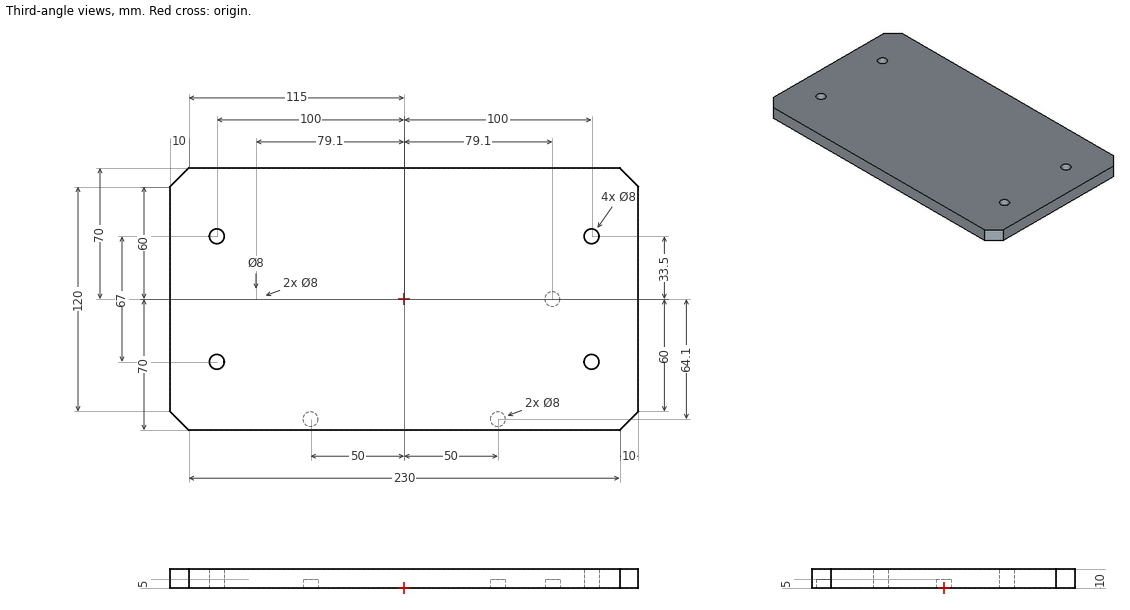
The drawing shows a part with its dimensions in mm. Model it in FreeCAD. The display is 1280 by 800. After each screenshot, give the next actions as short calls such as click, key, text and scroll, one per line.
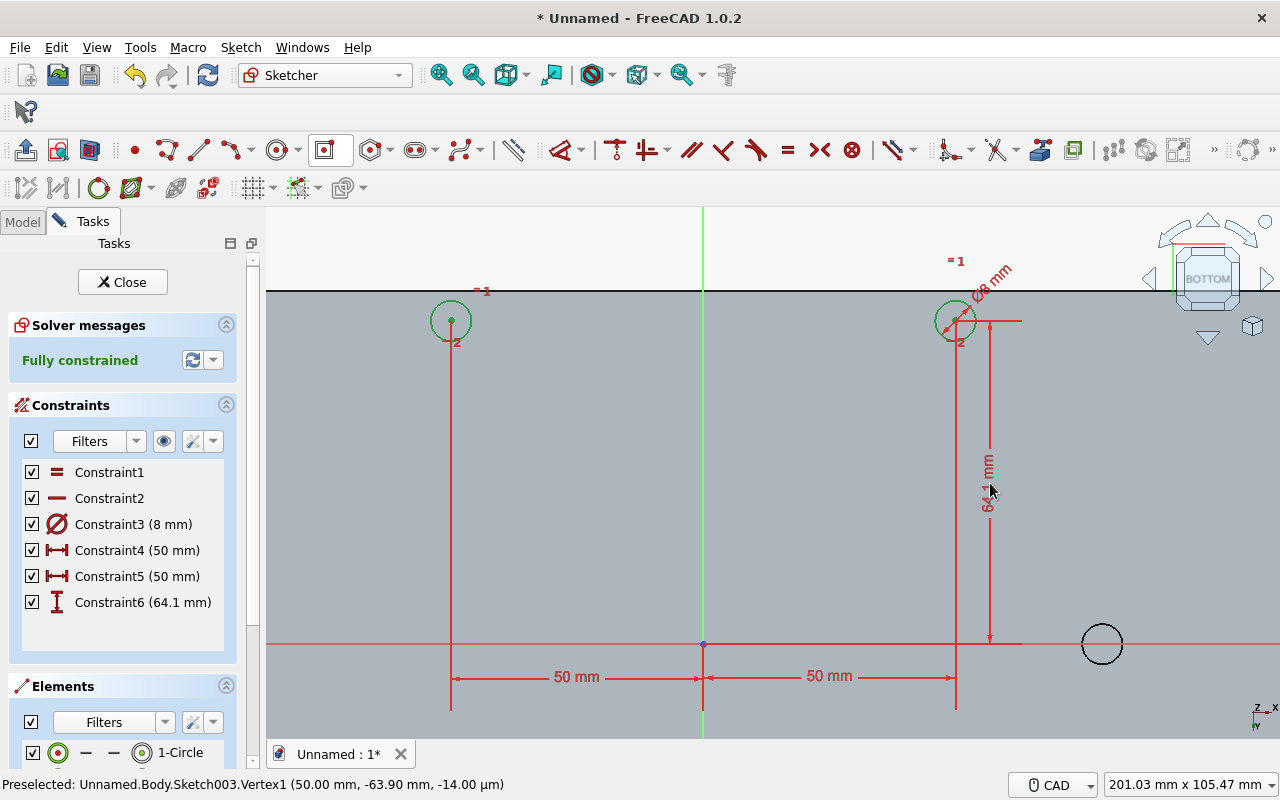
click(123, 282)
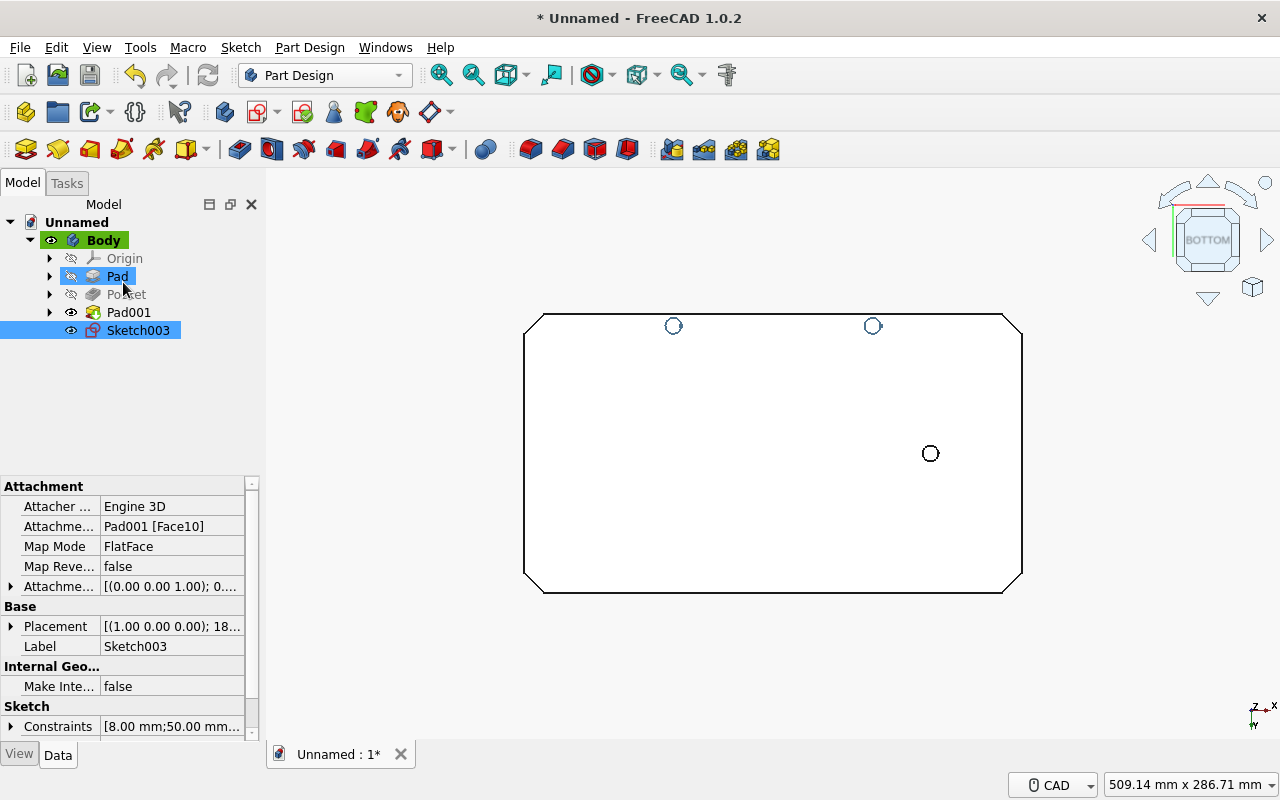
click(240, 150)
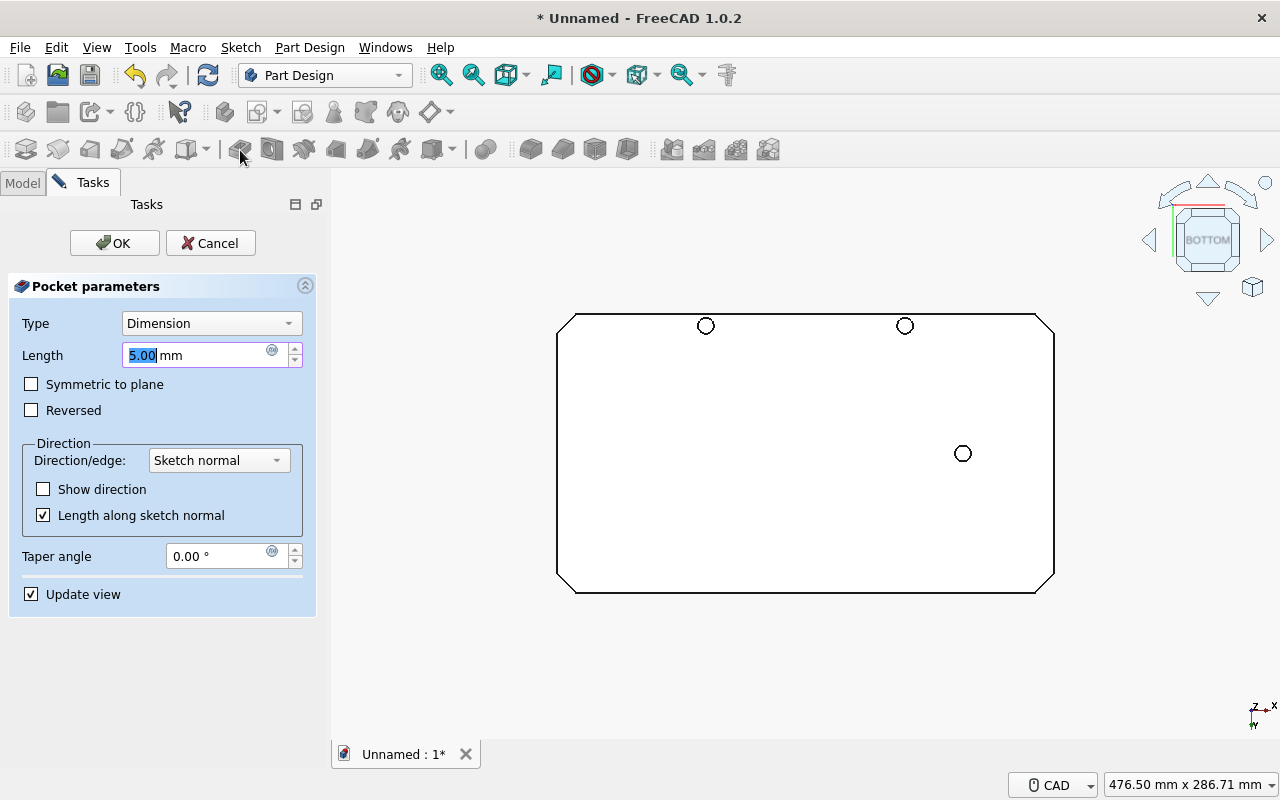
text(5)
key(Tab)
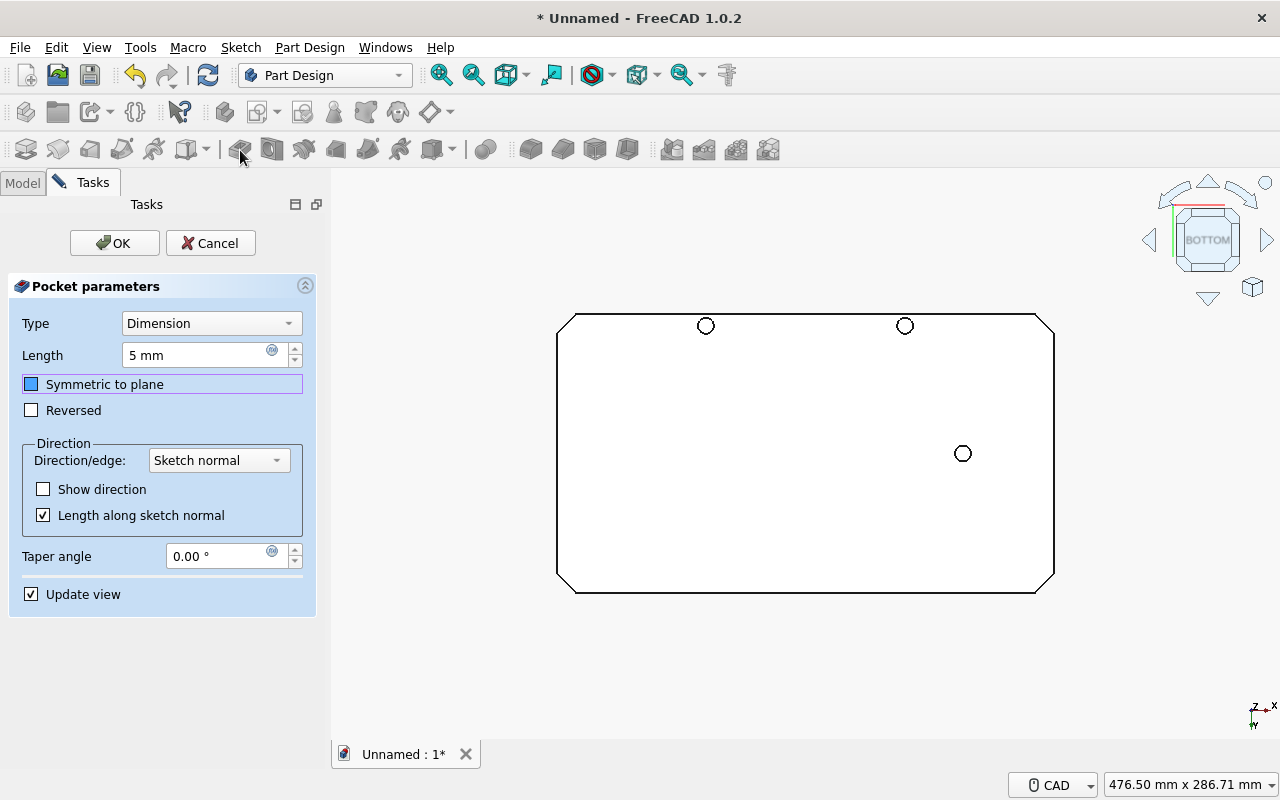
click(115, 243)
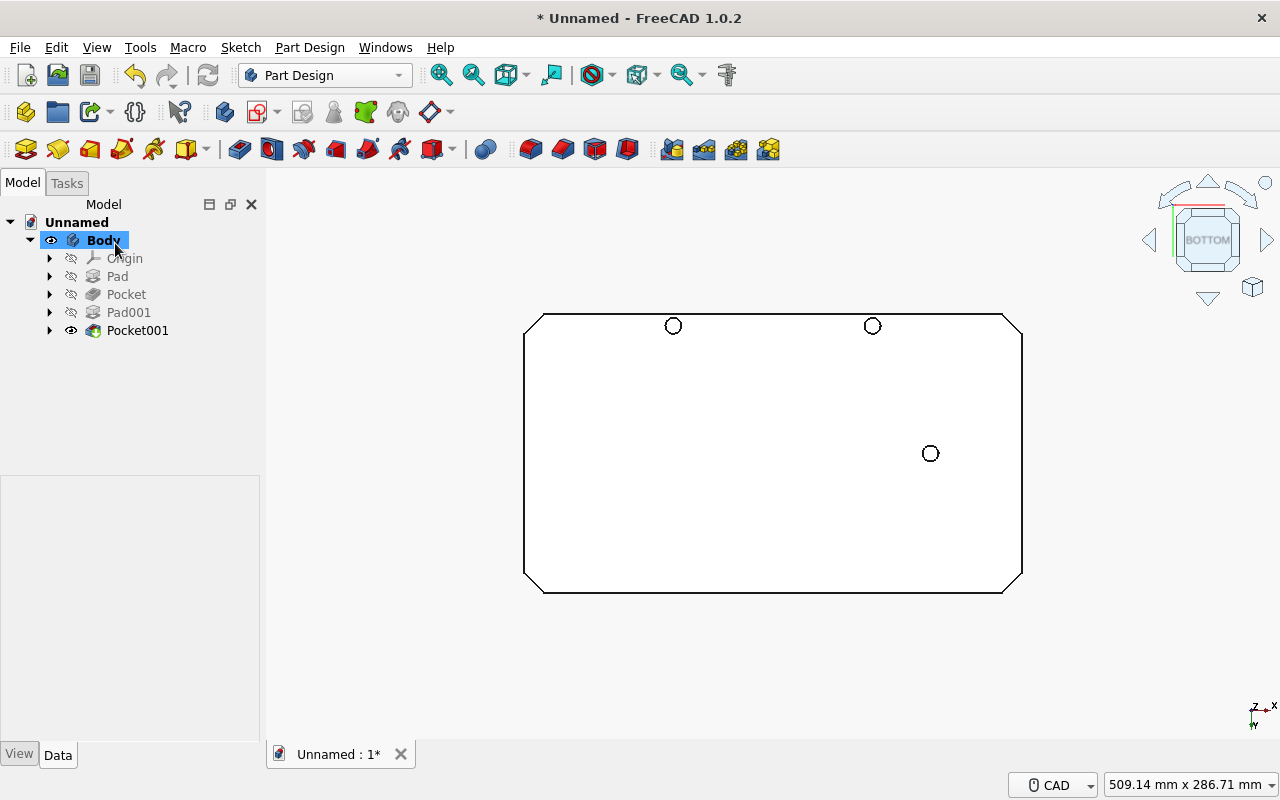
key(0)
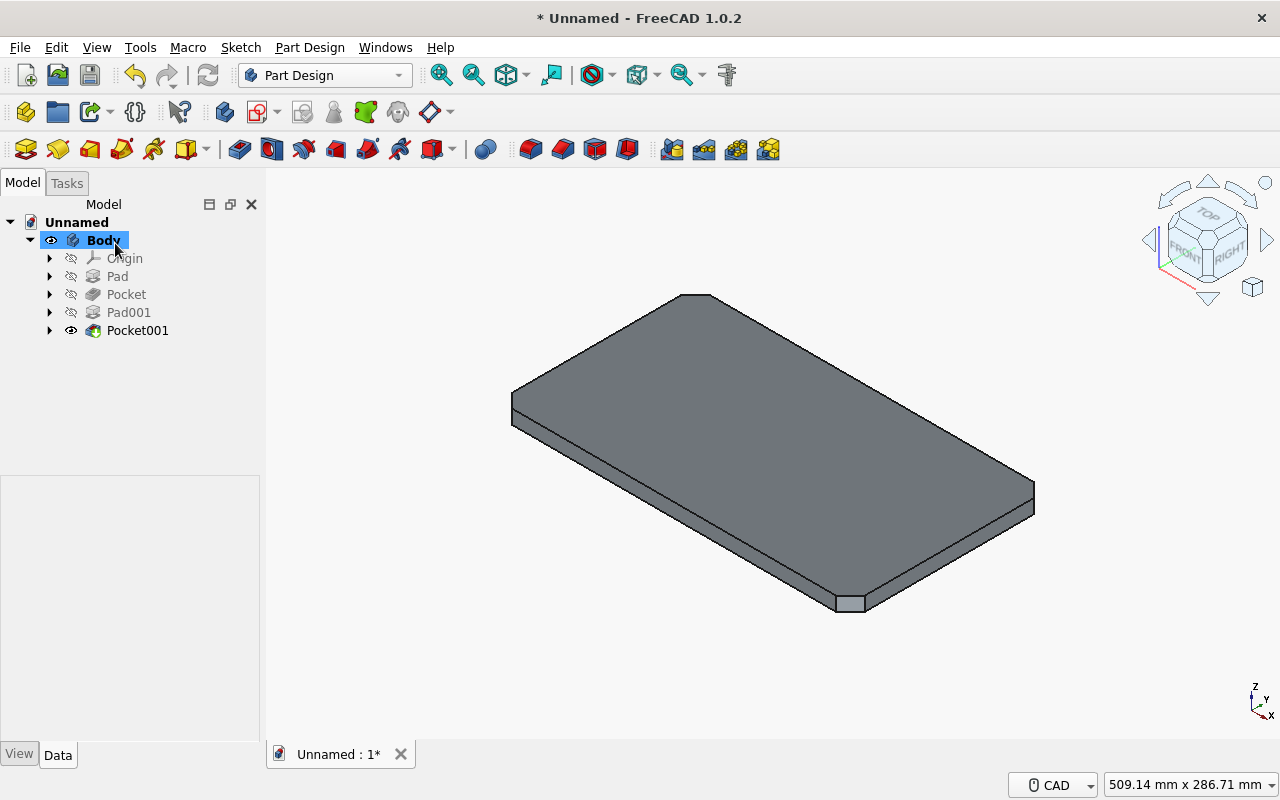
click(823, 473)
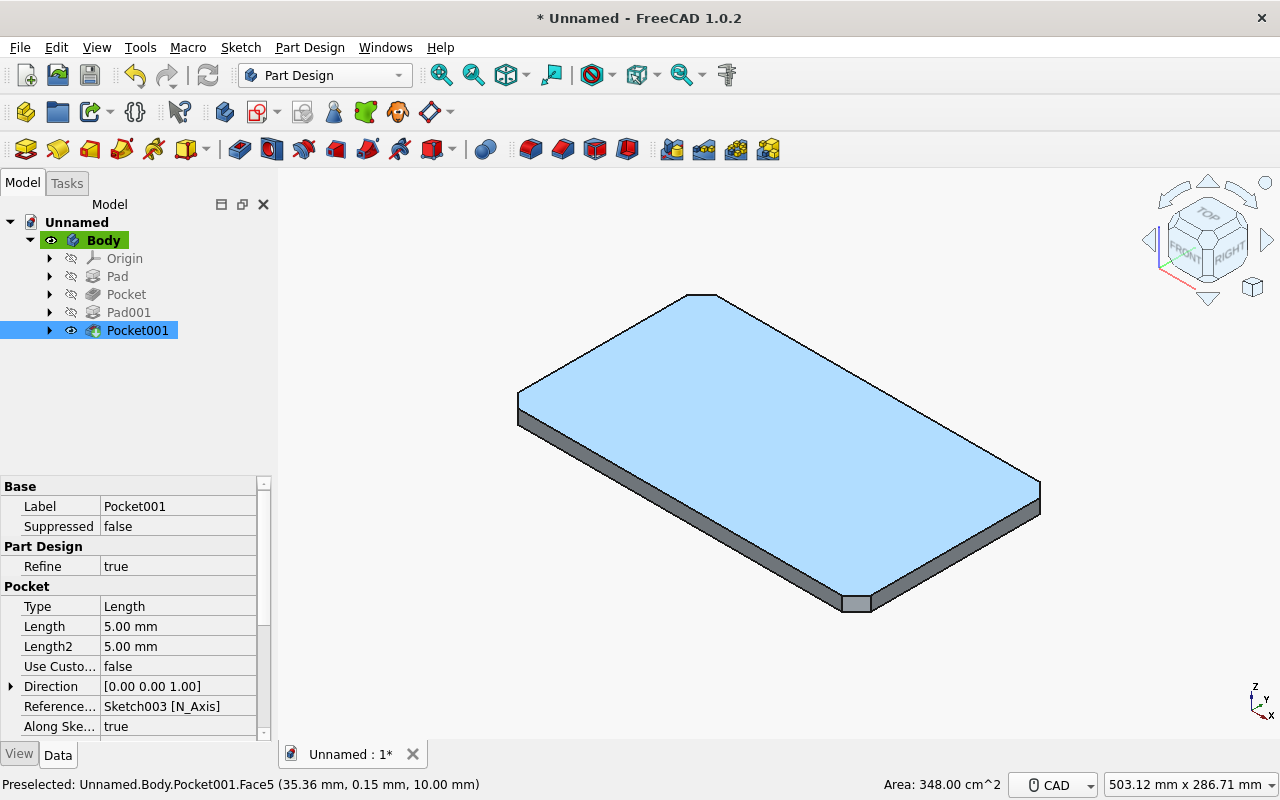
click(258, 112)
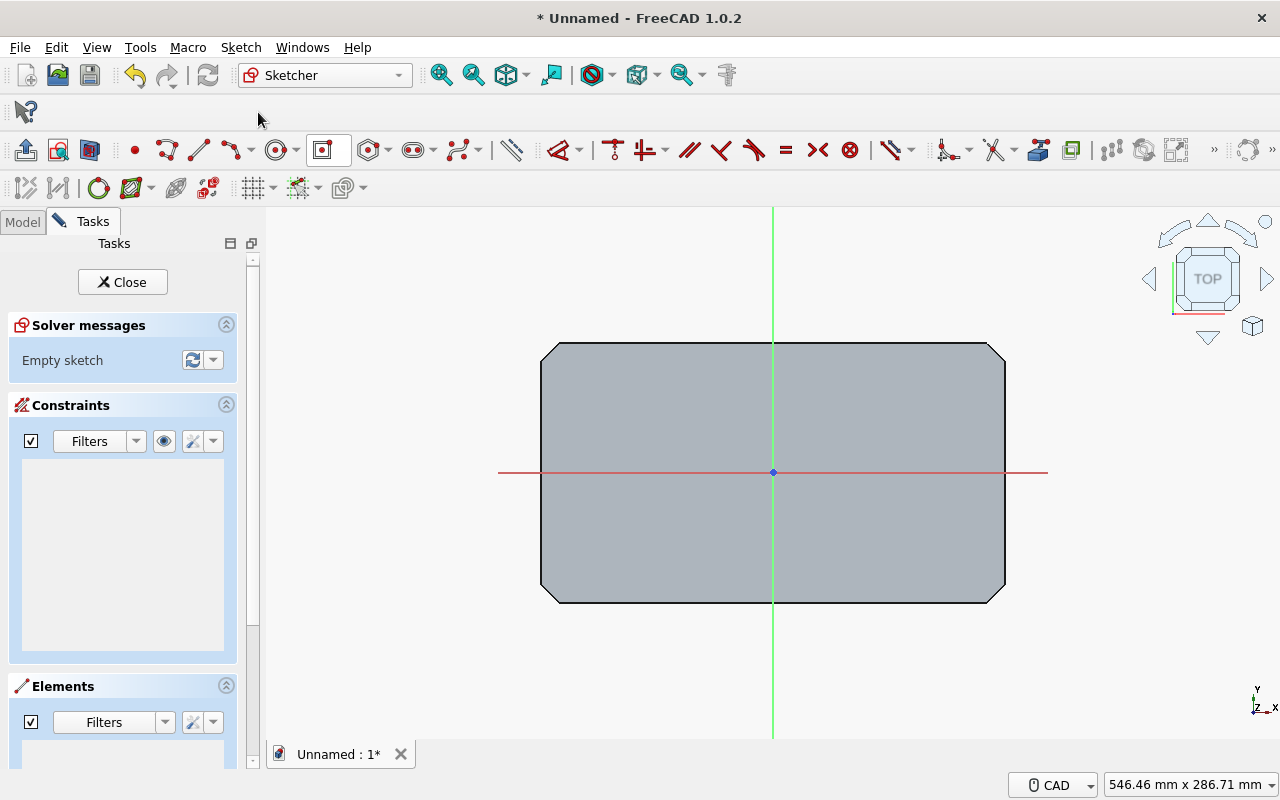
scroll(912, 473, up, 2)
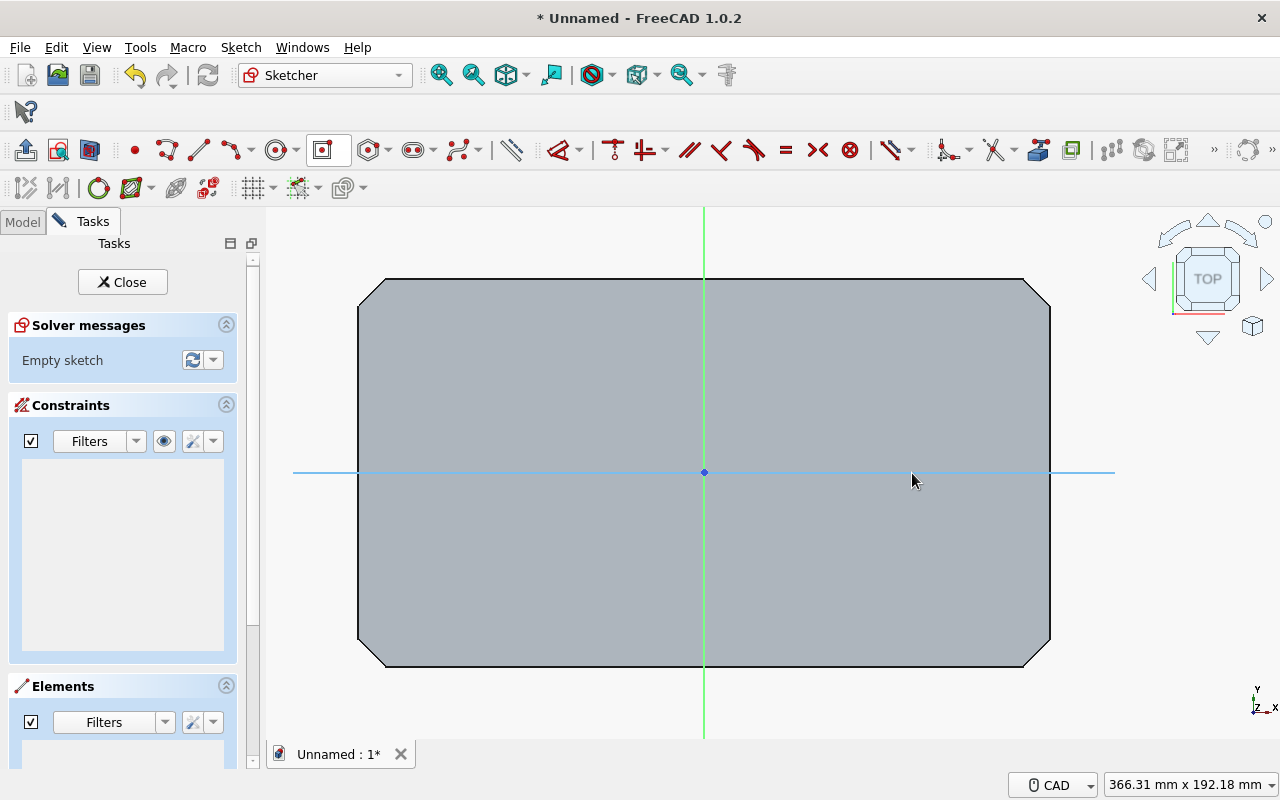
click(276, 150)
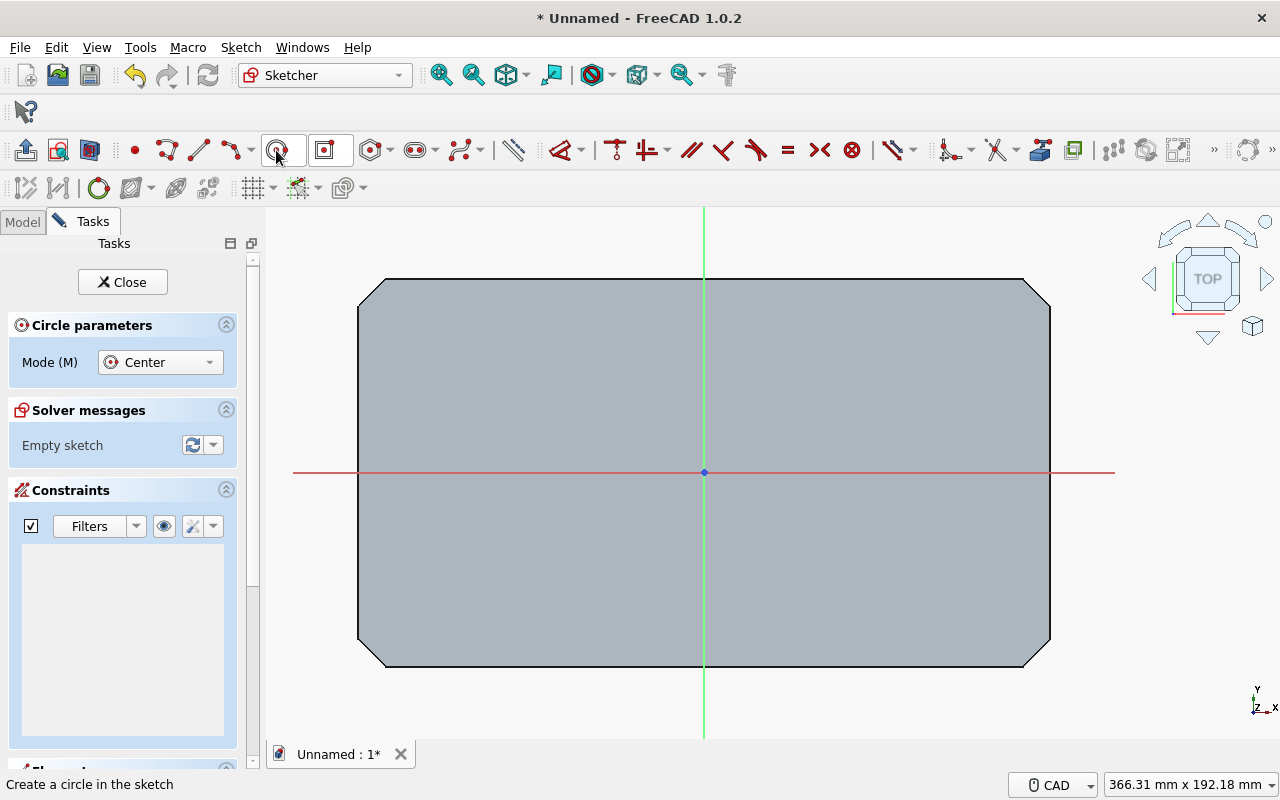
scroll(981, 380, up, 4)